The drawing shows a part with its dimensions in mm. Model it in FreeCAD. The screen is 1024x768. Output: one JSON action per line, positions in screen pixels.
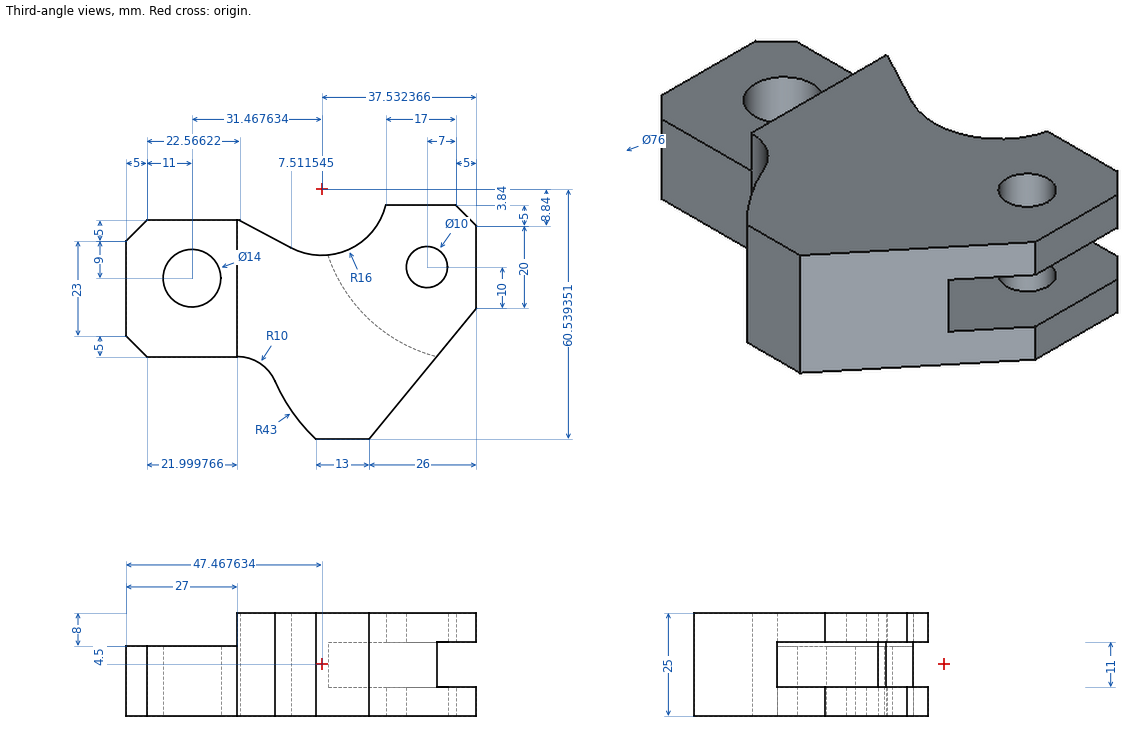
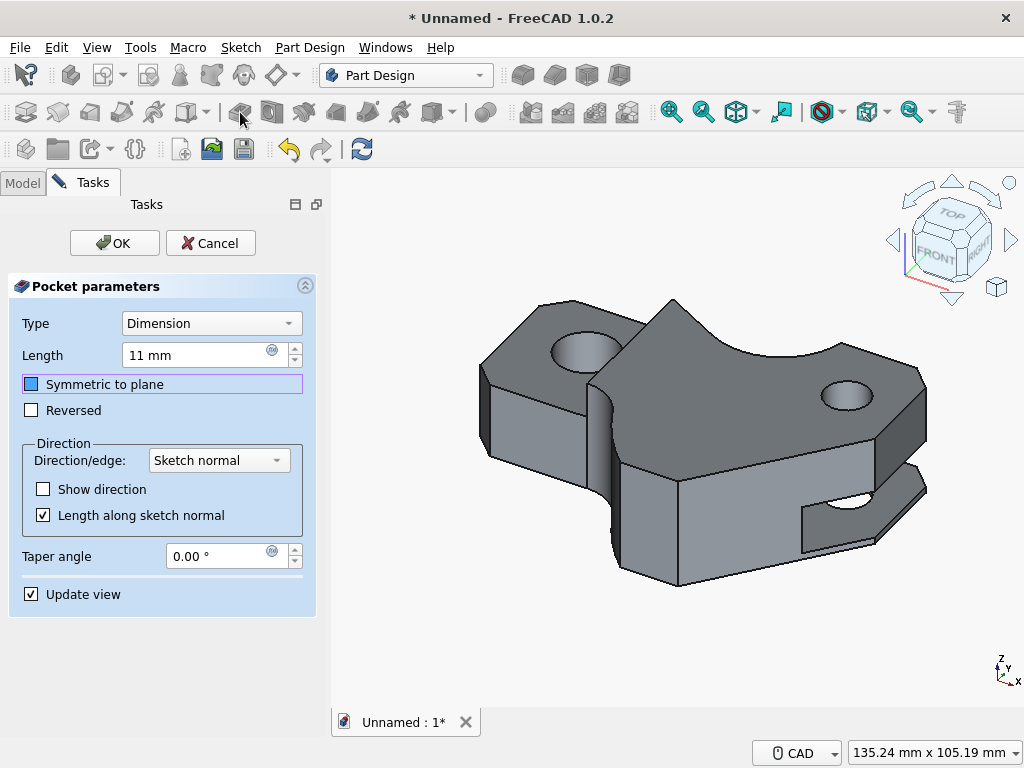
{"action": "left_click", "coordinate": [30, 384]}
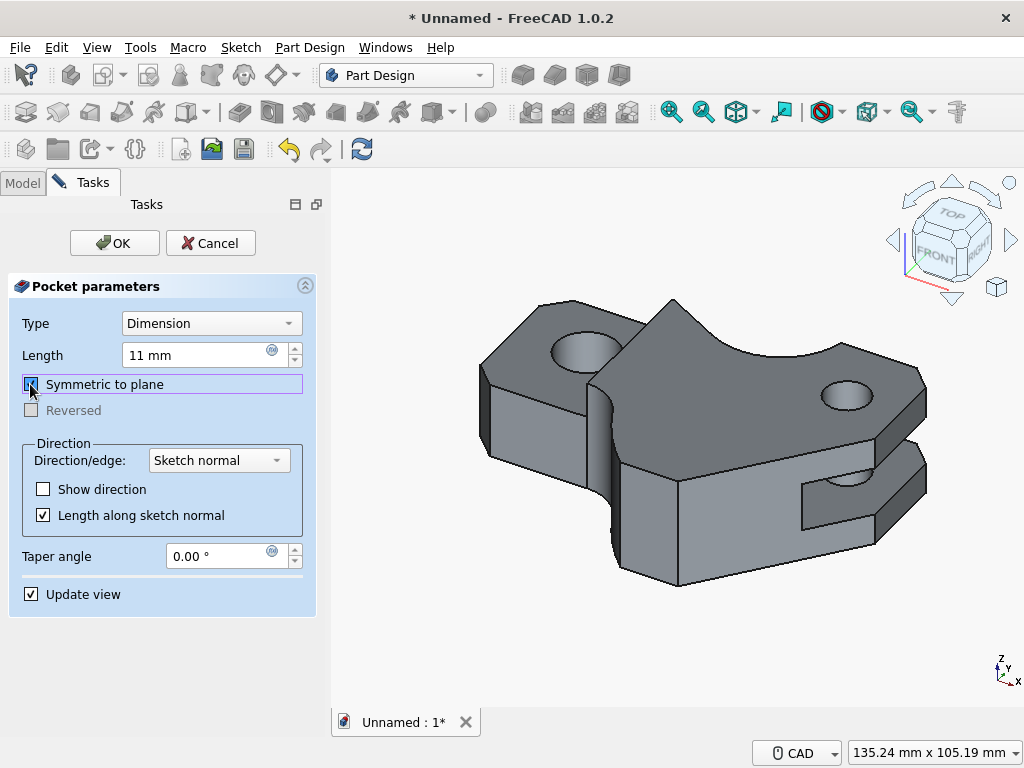
{"action": "left_click", "coordinate": [115, 243]}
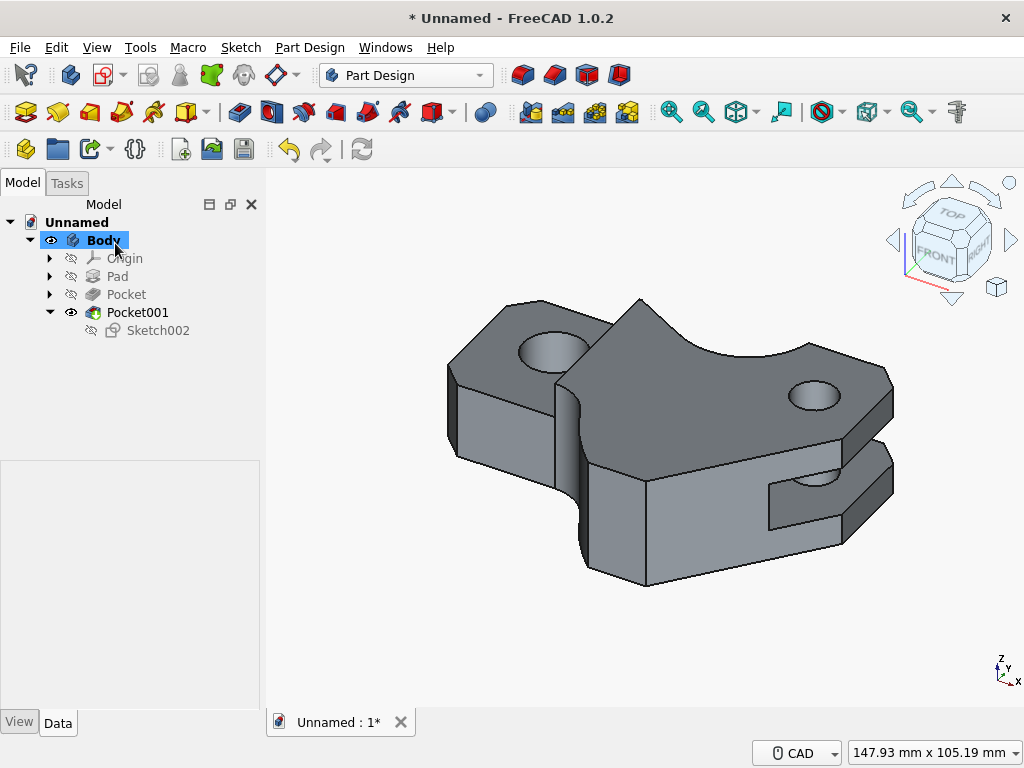
{"action": "key", "text": "0"}